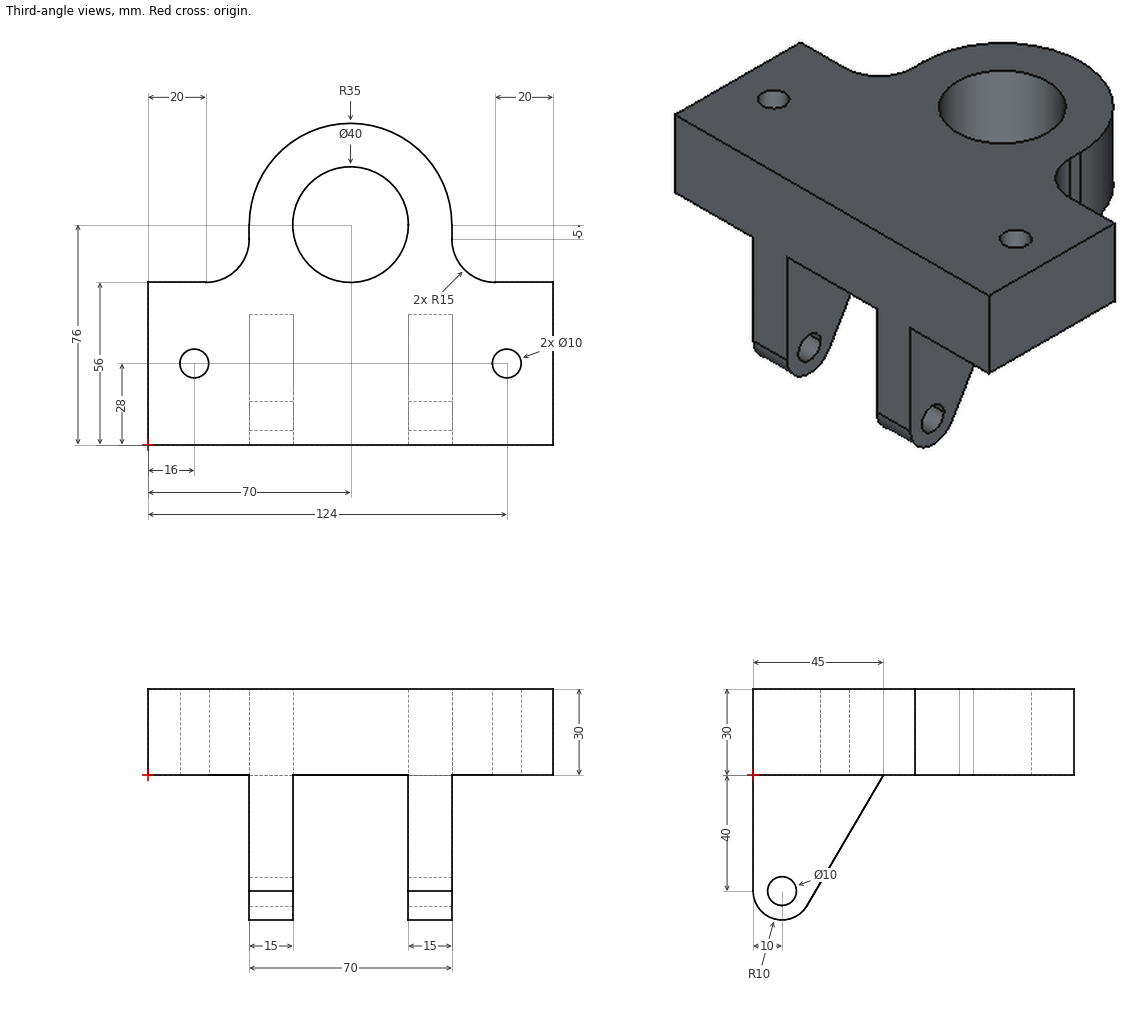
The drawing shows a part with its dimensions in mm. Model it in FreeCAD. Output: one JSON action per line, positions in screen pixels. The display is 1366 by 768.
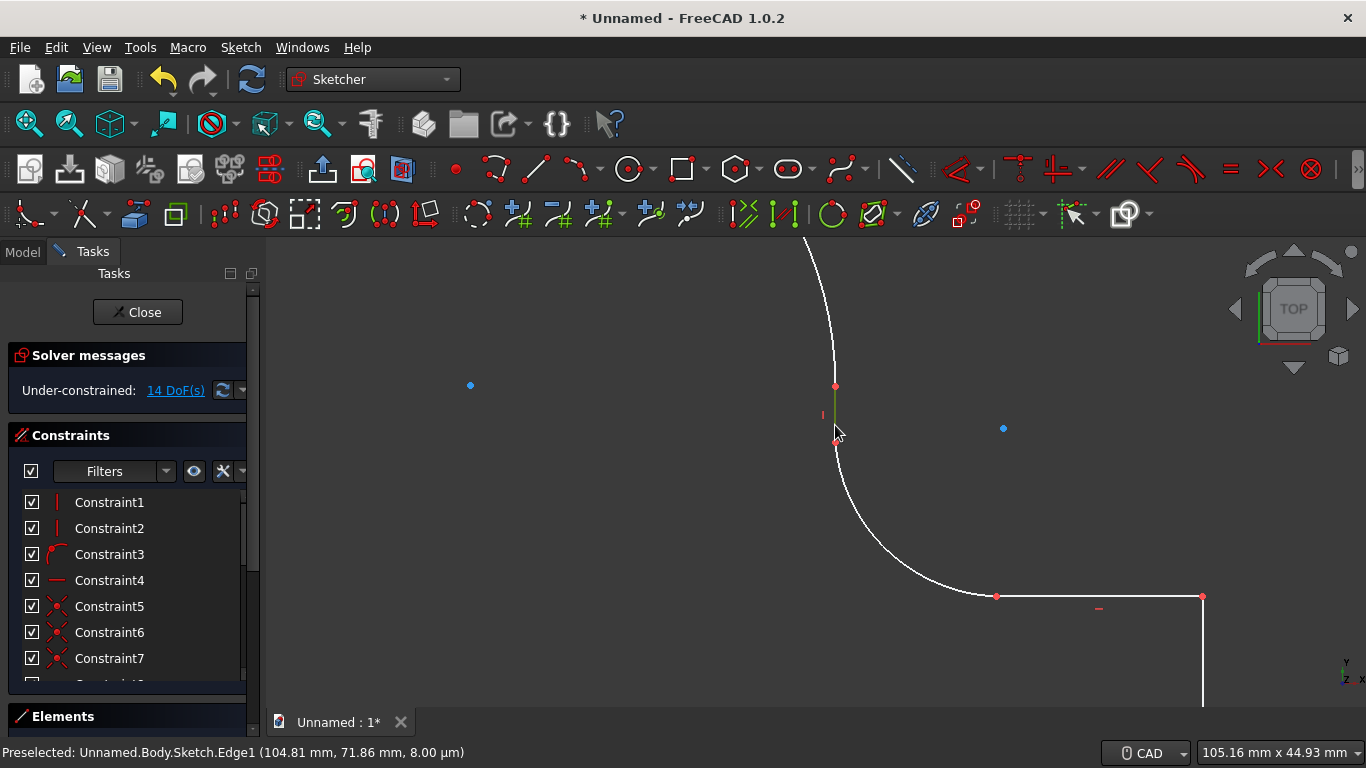
{"action": "scroll", "coordinate": [838, 431], "scroll_direction": "down", "scroll_amount": 7}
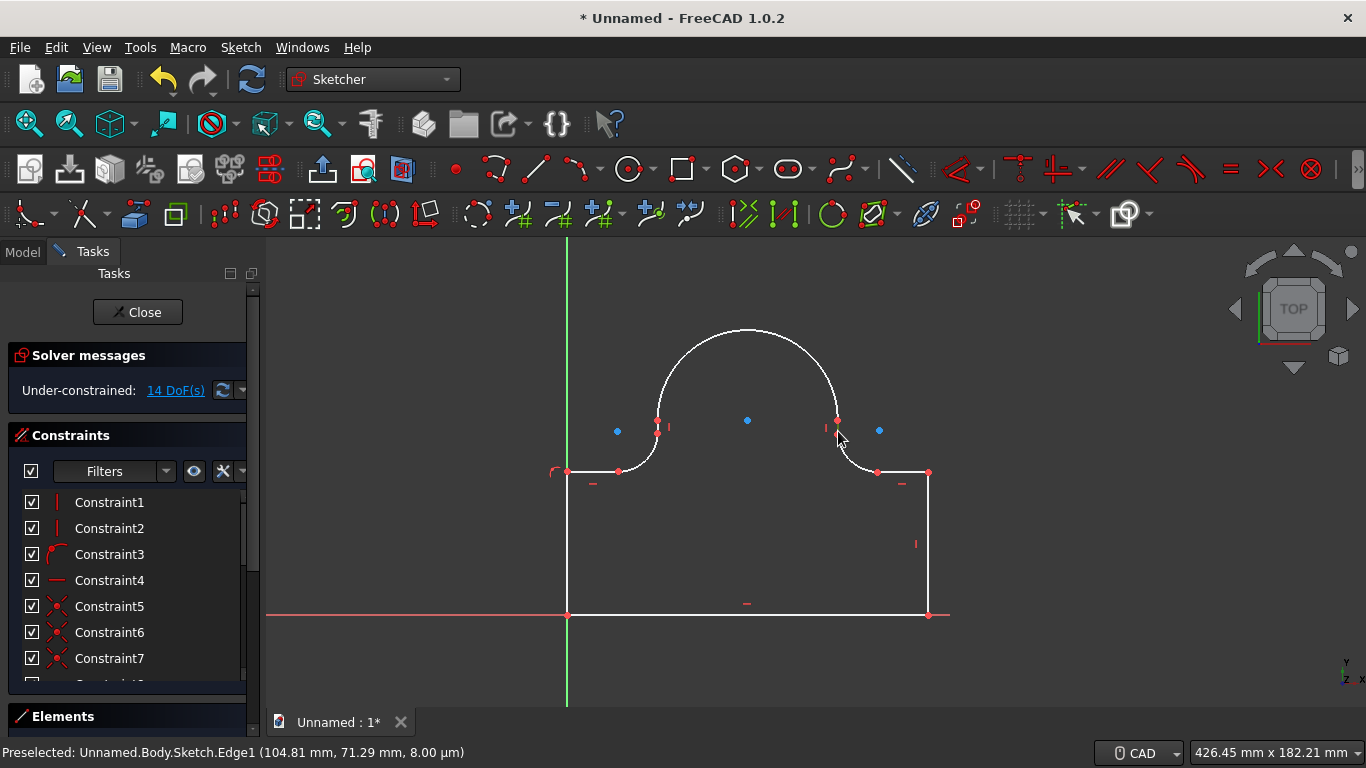
{"action": "left_click", "coordinate": [801, 347]}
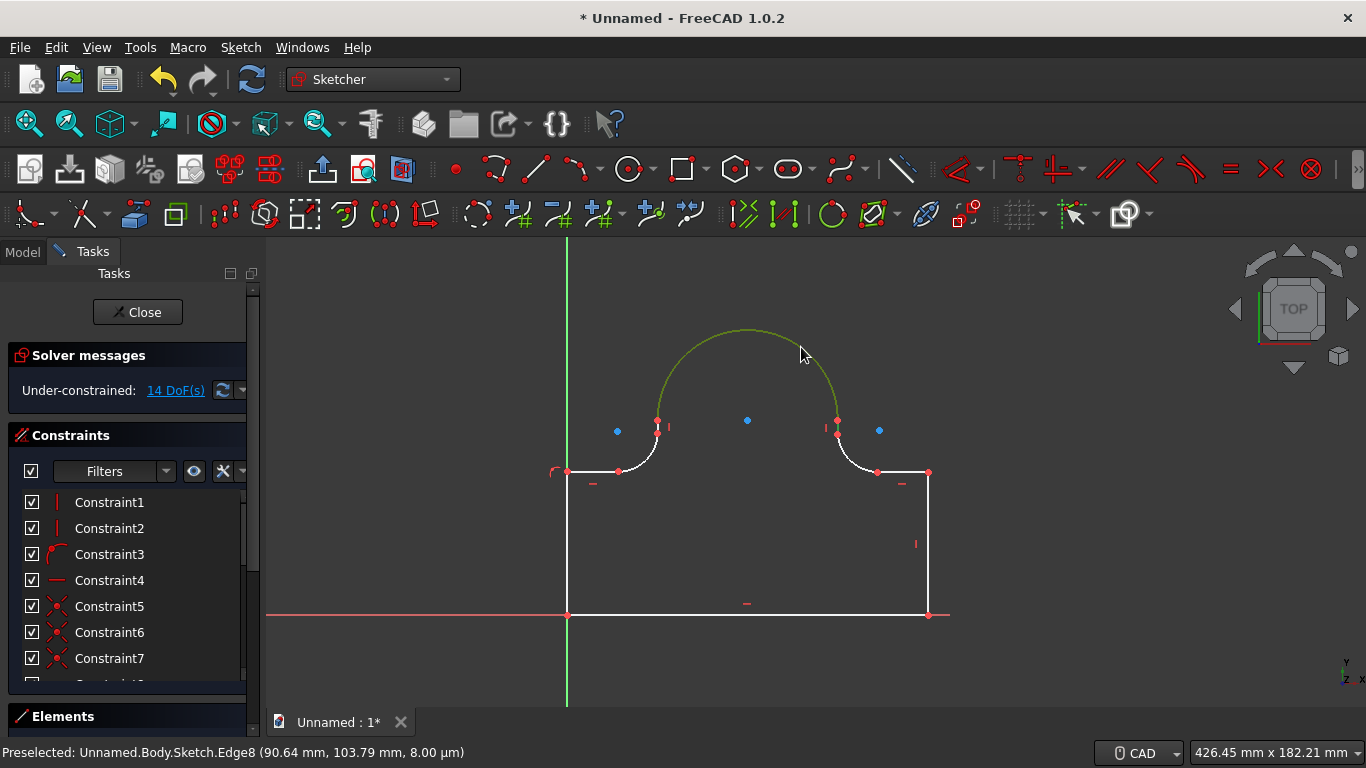
{"action": "left_click", "coordinate": [1192, 170]}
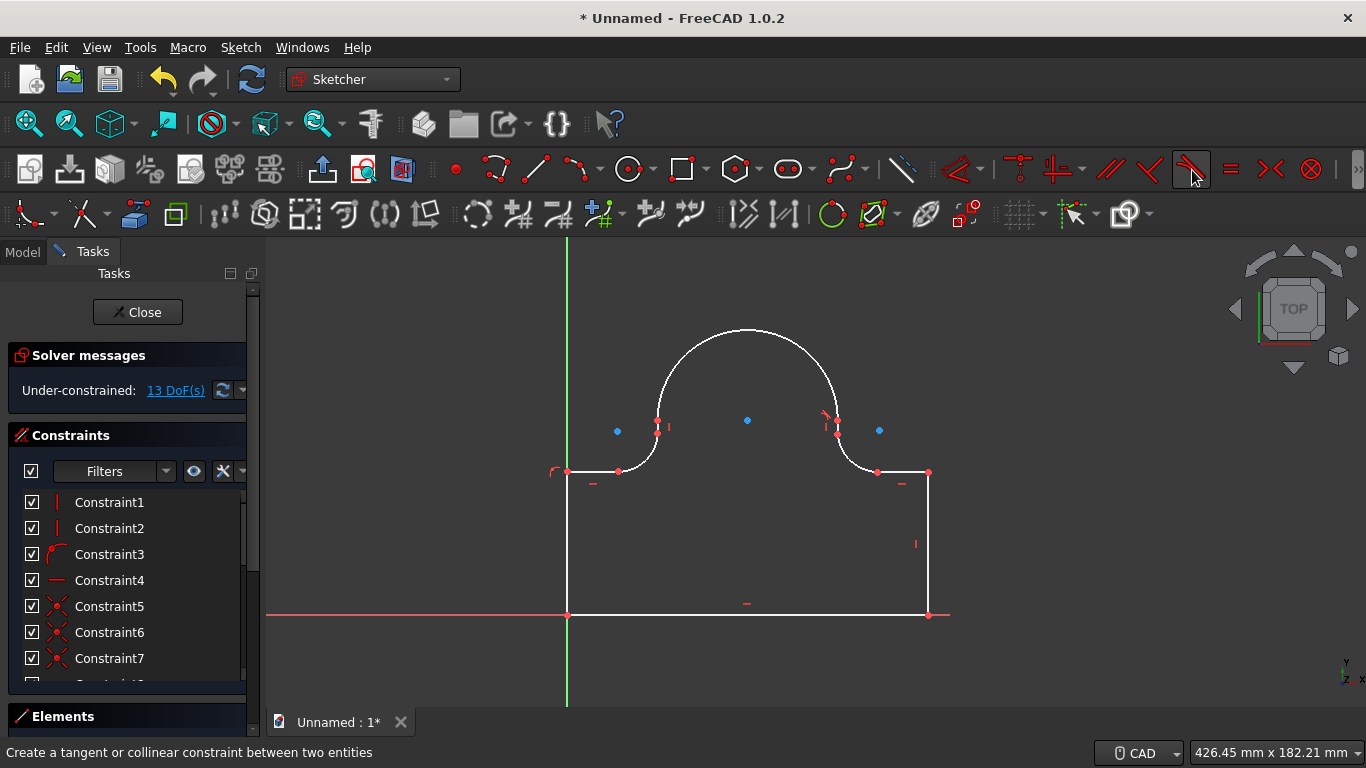
{"action": "scroll", "coordinate": [838, 427], "scroll_direction": "up", "scroll_amount": 4}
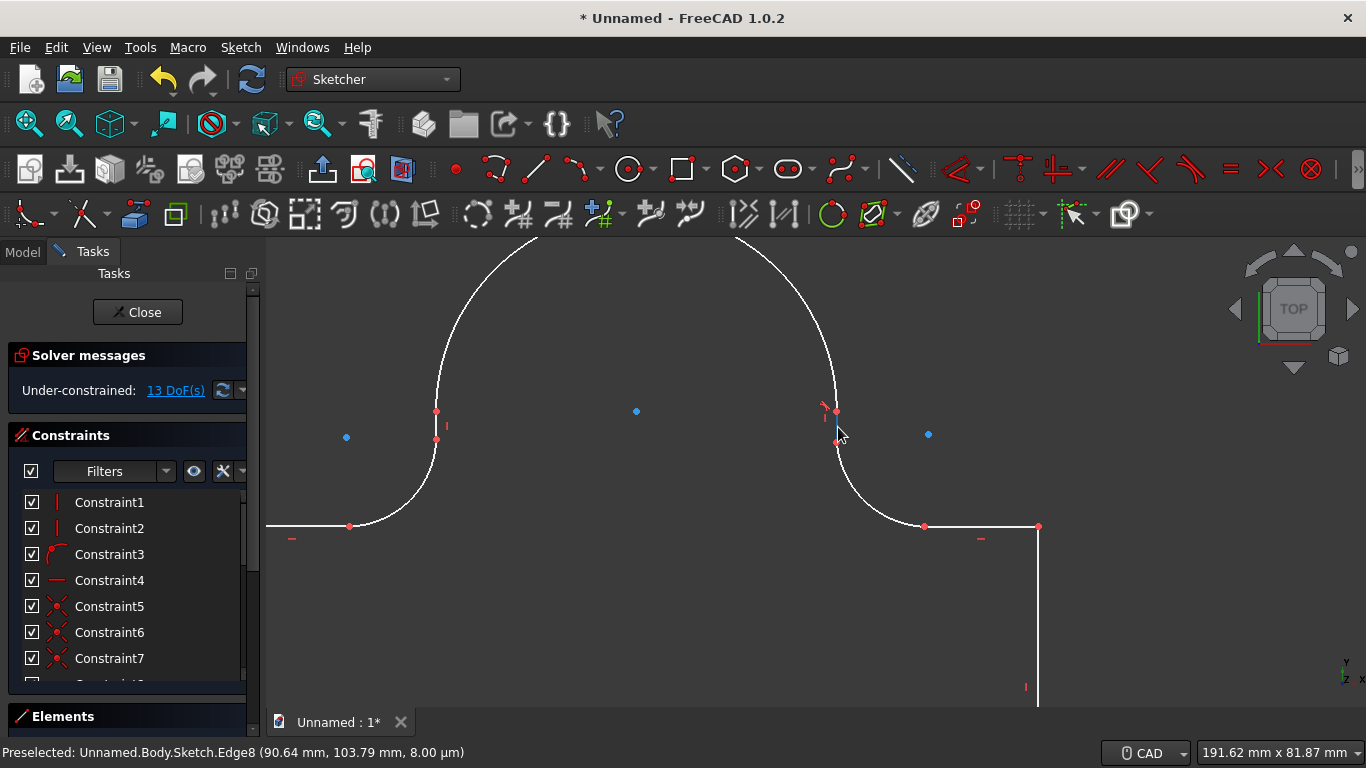
{"action": "left_click", "coordinate": [837, 427]}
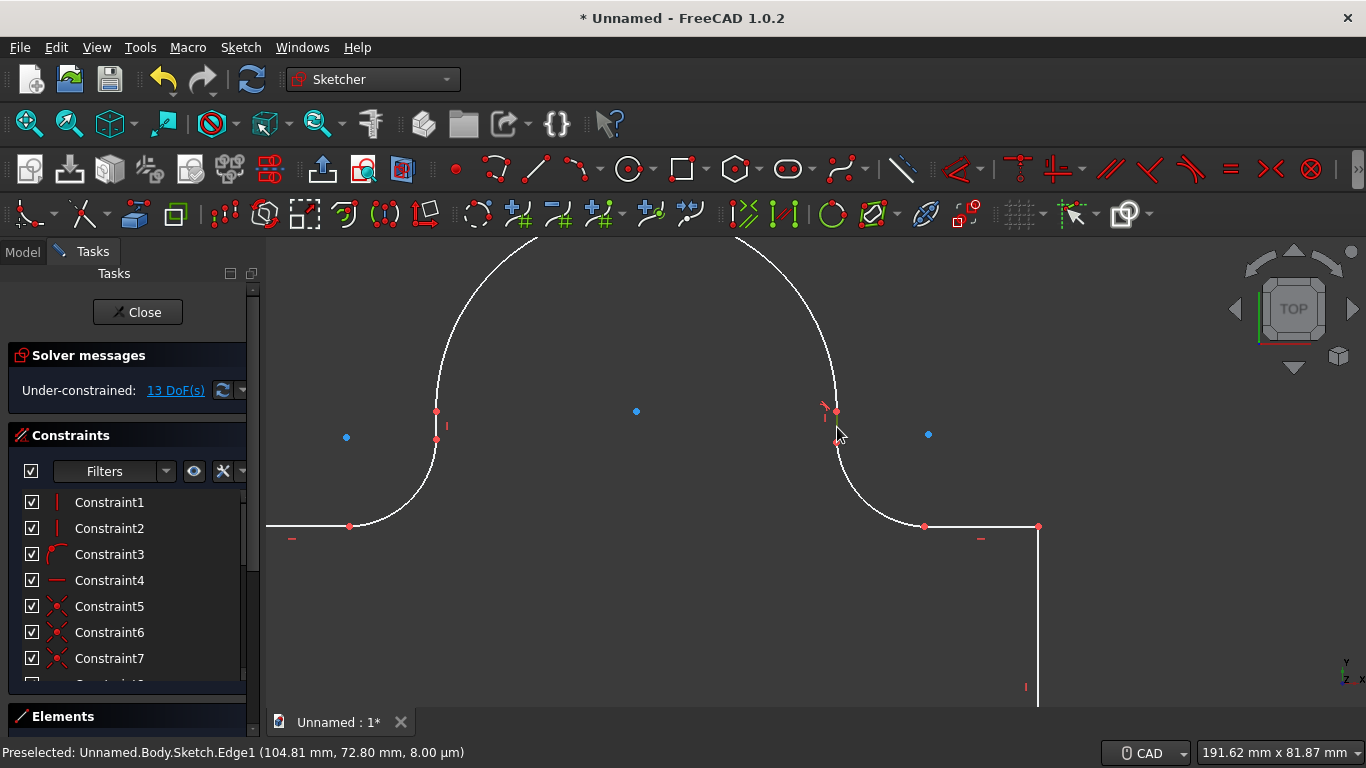
{"action": "left_click", "coordinate": [849, 480]}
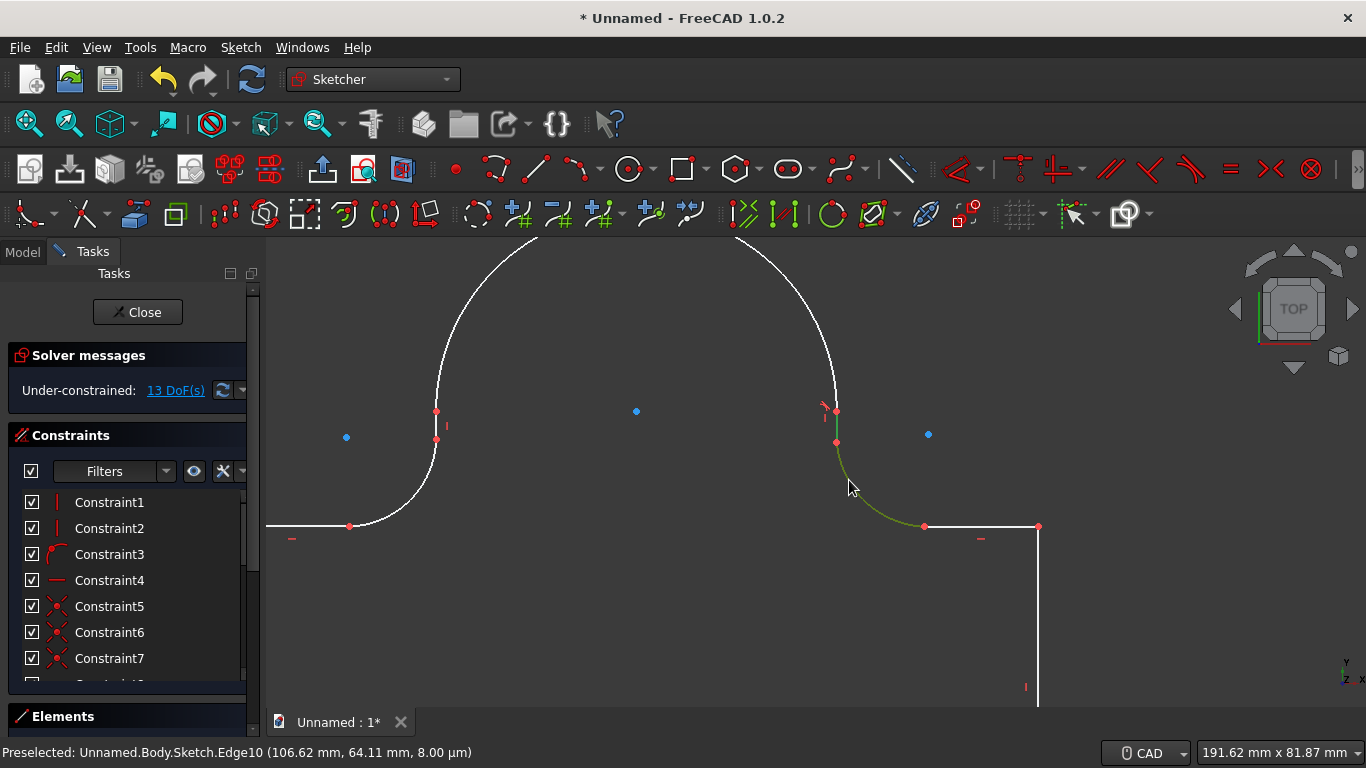
{"action": "key", "text": "t"}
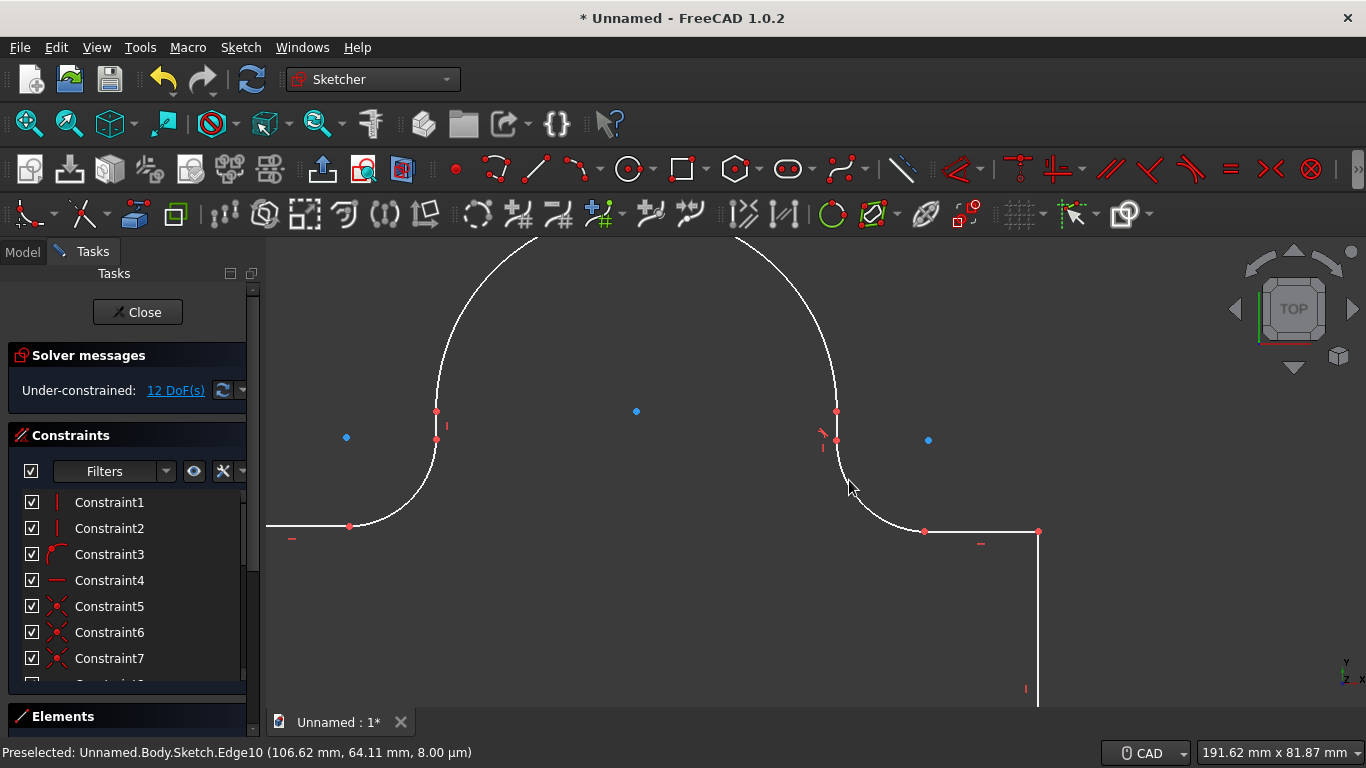
{"action": "left_click", "coordinate": [436, 423]}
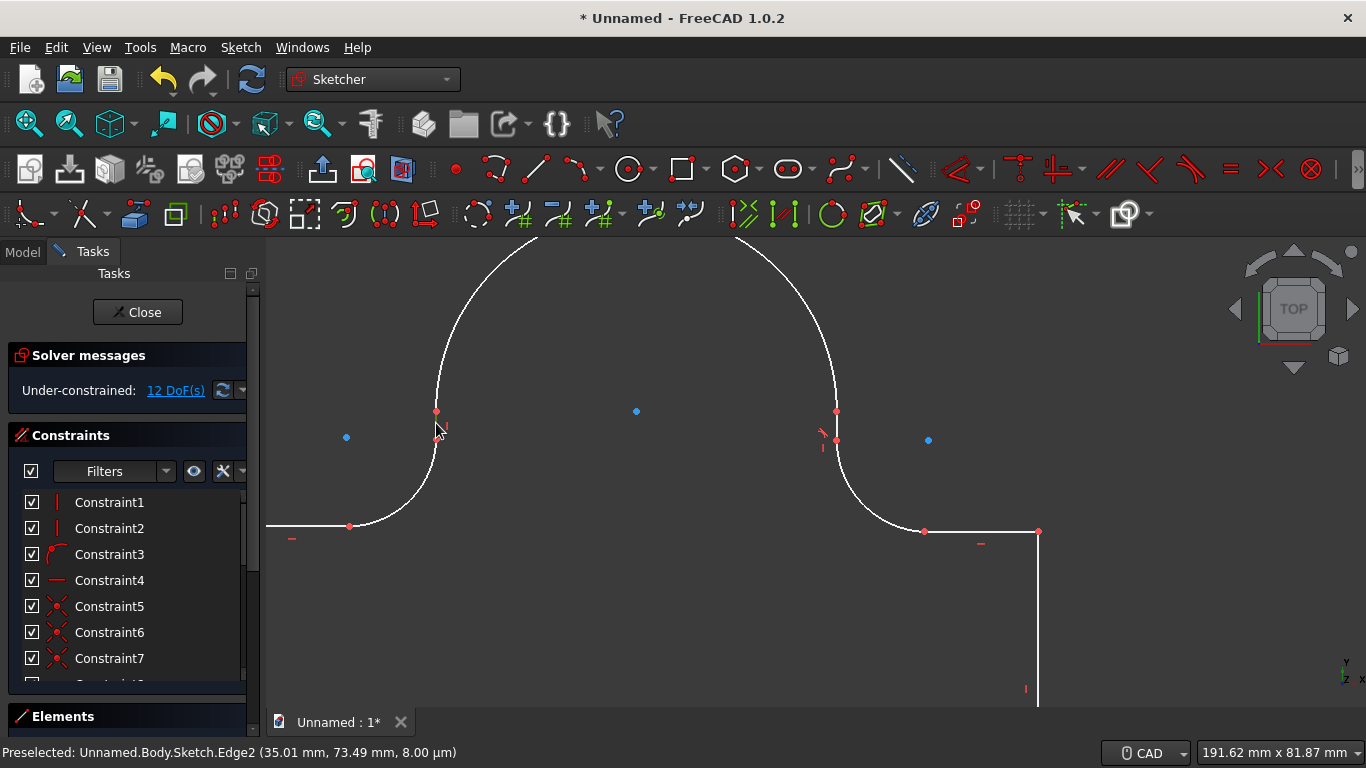
{"action": "left_click", "coordinate": [799, 293]}